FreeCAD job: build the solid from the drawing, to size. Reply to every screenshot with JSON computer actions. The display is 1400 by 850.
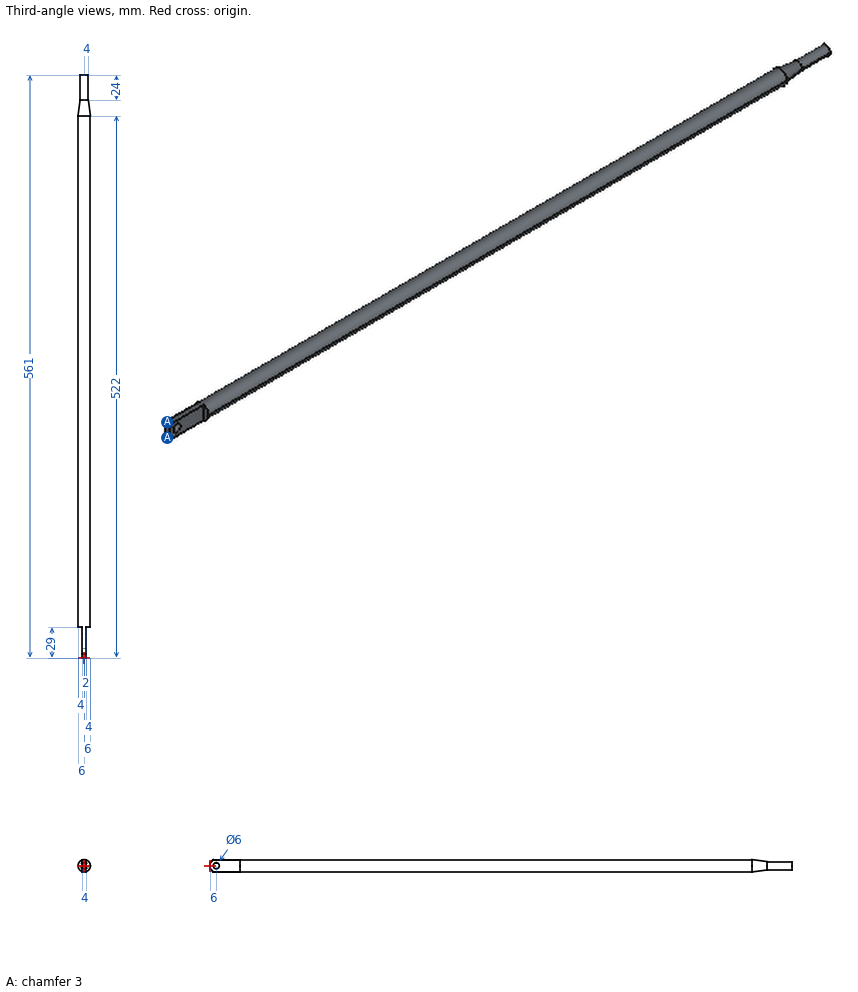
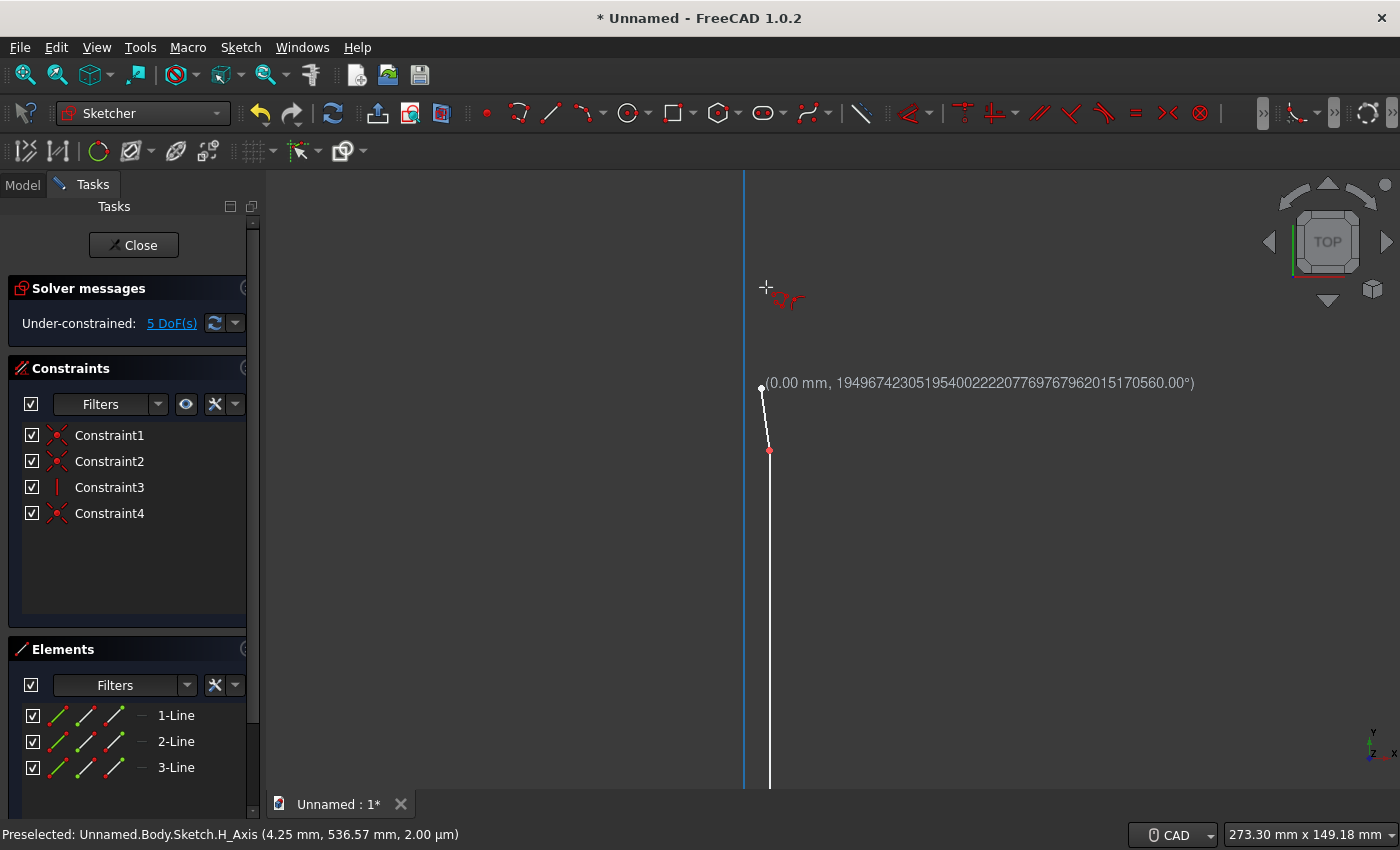
{"action": "left_click", "coordinate": [761, 288]}
{"action": "left_click", "coordinate": [753, 288]}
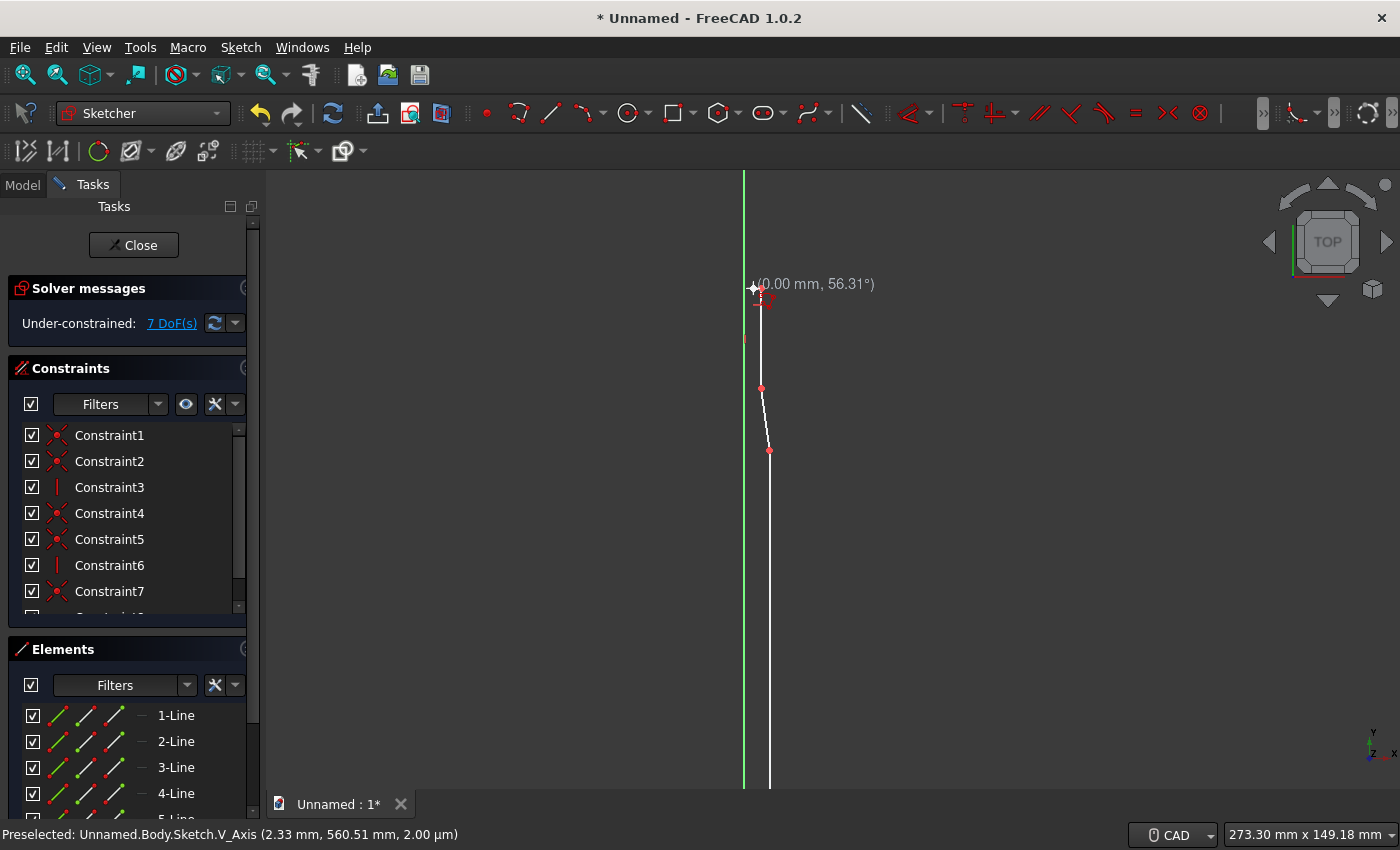
{"action": "scroll", "coordinate": [766, 287], "scroll_direction": "down", "scroll_amount": 9}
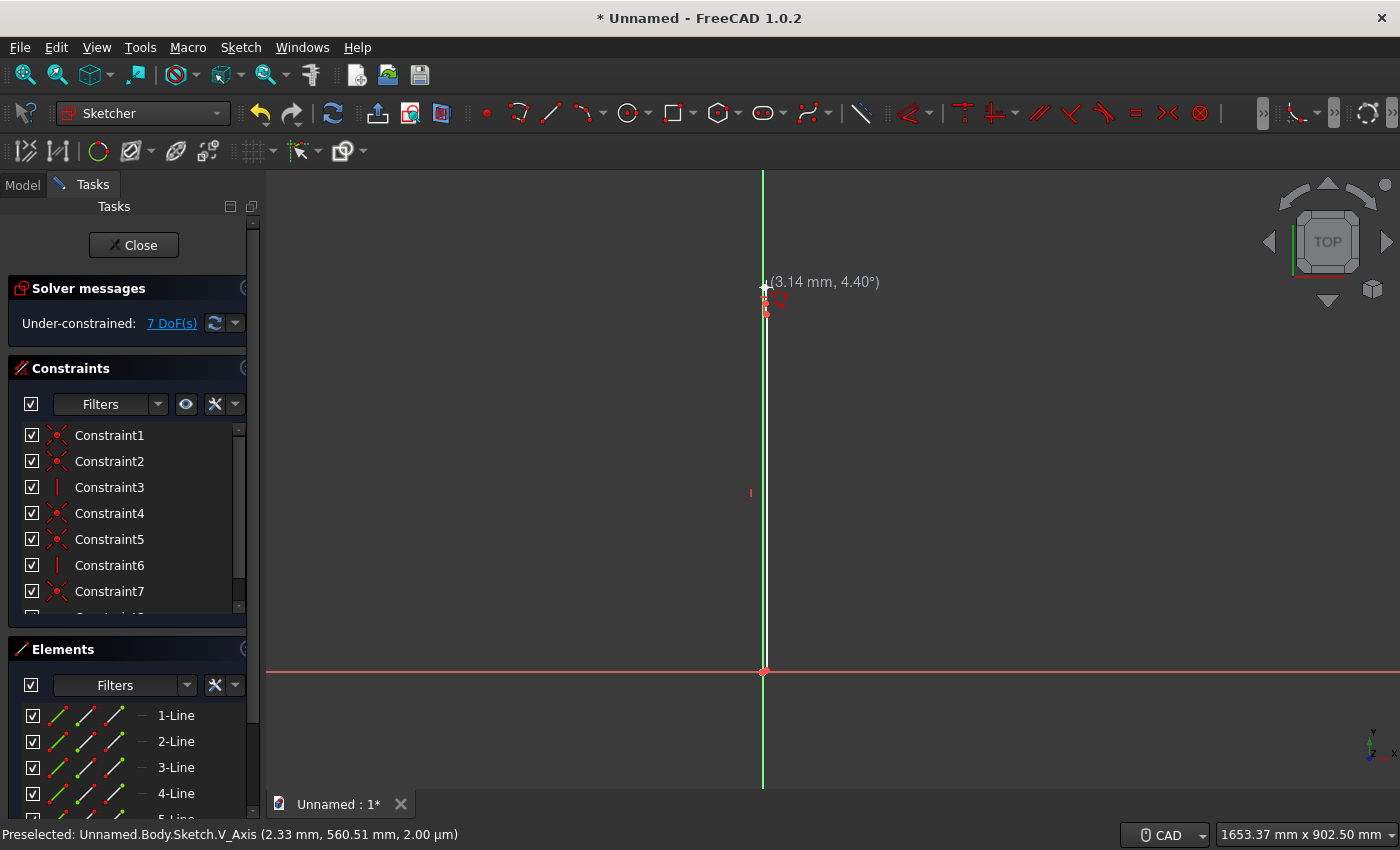
{"action": "scroll", "coordinate": [763, 672], "scroll_direction": "up", "scroll_amount": 11}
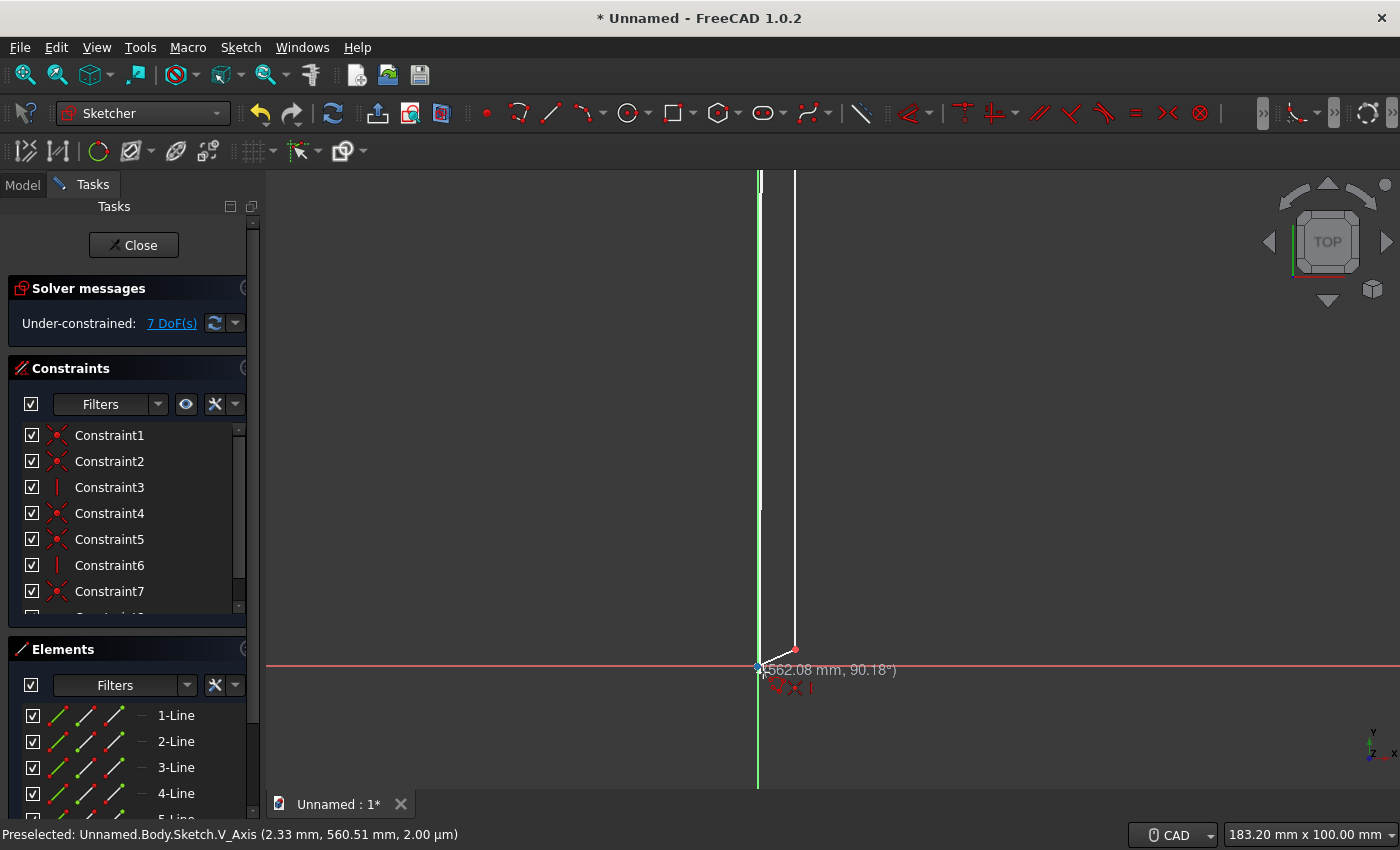
{"action": "left_click", "coordinate": [758, 666]}
{"action": "key", "text": "Escape"}
{"action": "key", "text": "Escape"}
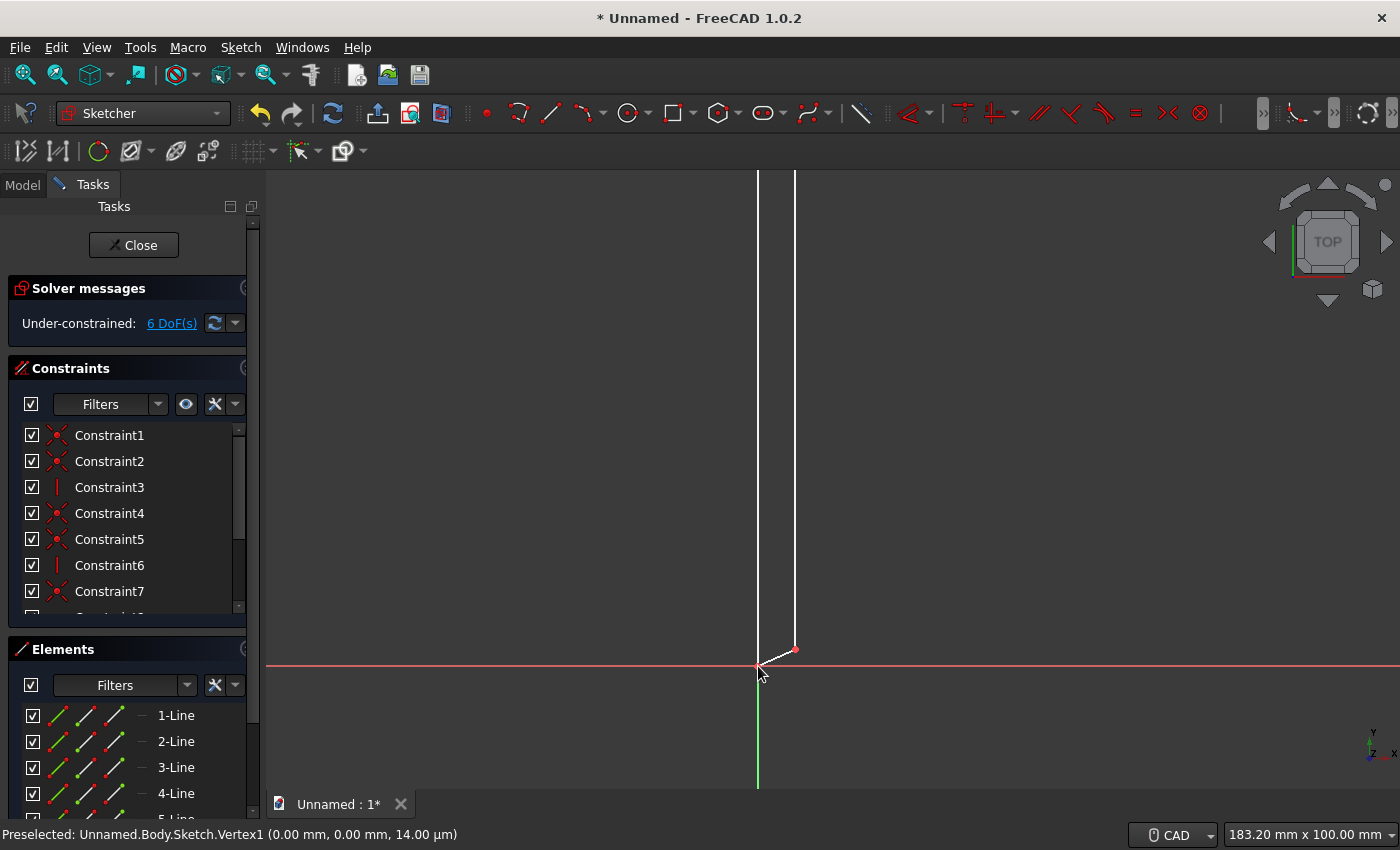
{"action": "left_click", "coordinate": [784, 654]}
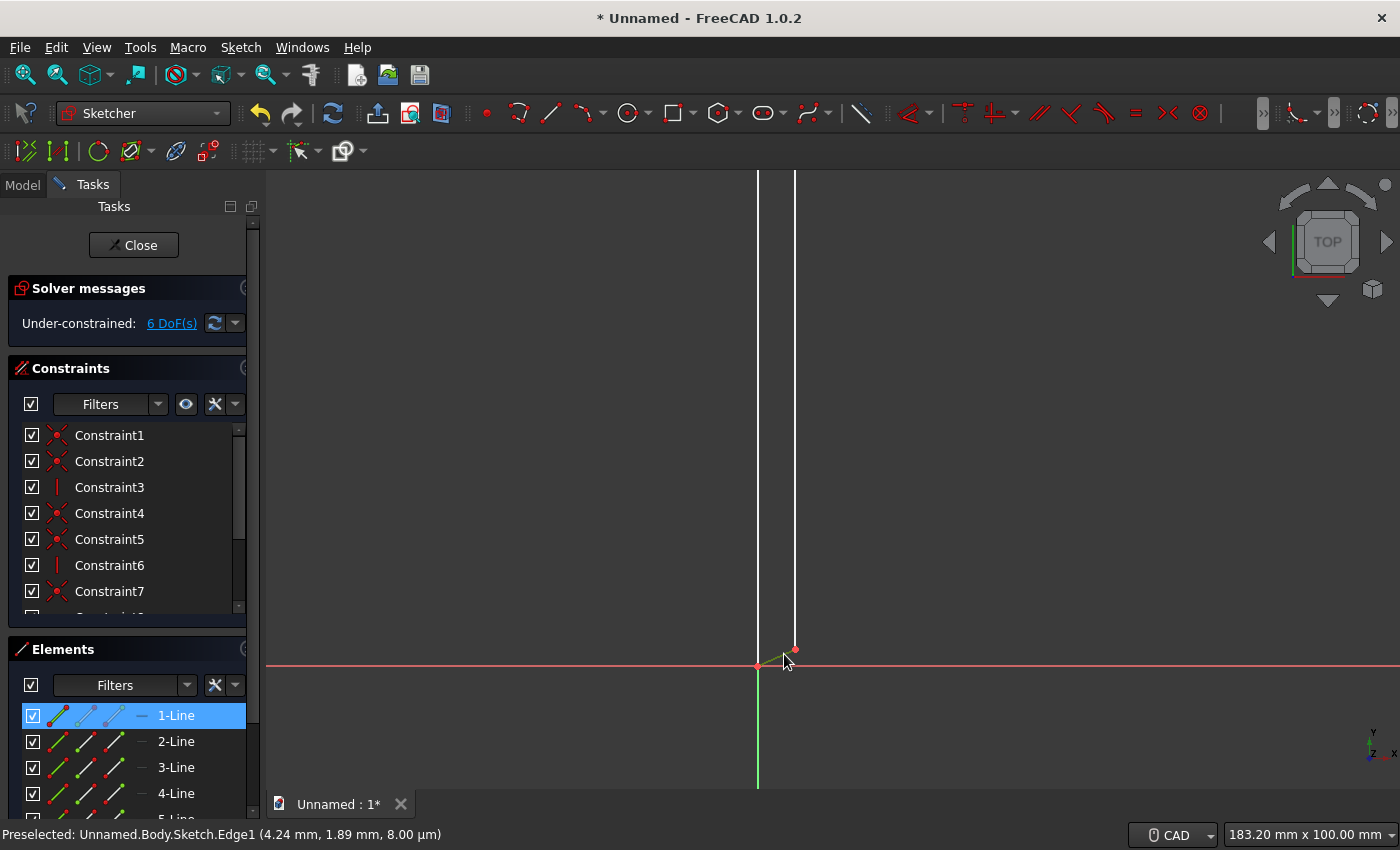
{"action": "left_click", "coordinate": [1018, 114]}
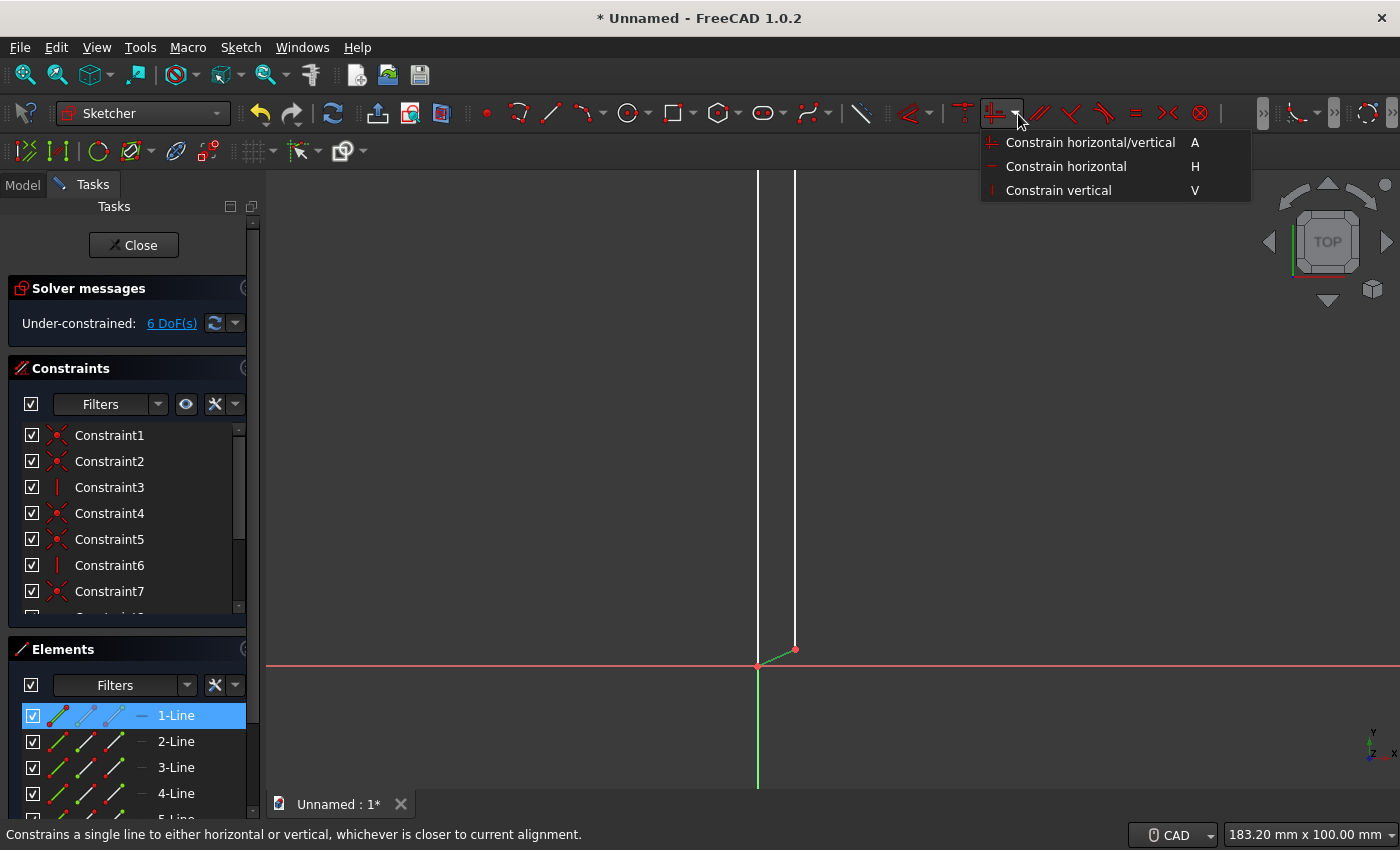
{"action": "left_click", "coordinate": [1116, 166]}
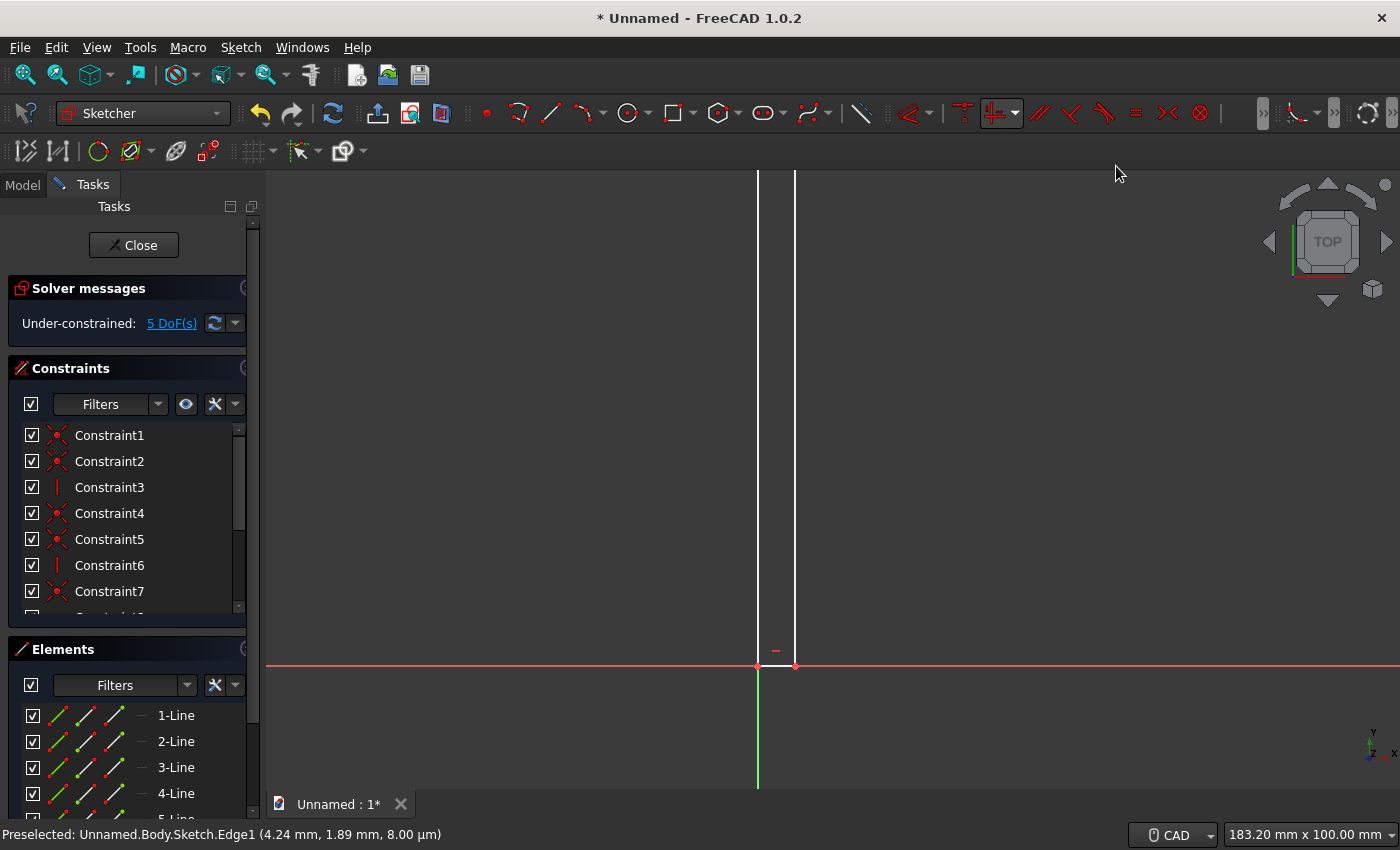
{"action": "left_click", "coordinate": [908, 114]}